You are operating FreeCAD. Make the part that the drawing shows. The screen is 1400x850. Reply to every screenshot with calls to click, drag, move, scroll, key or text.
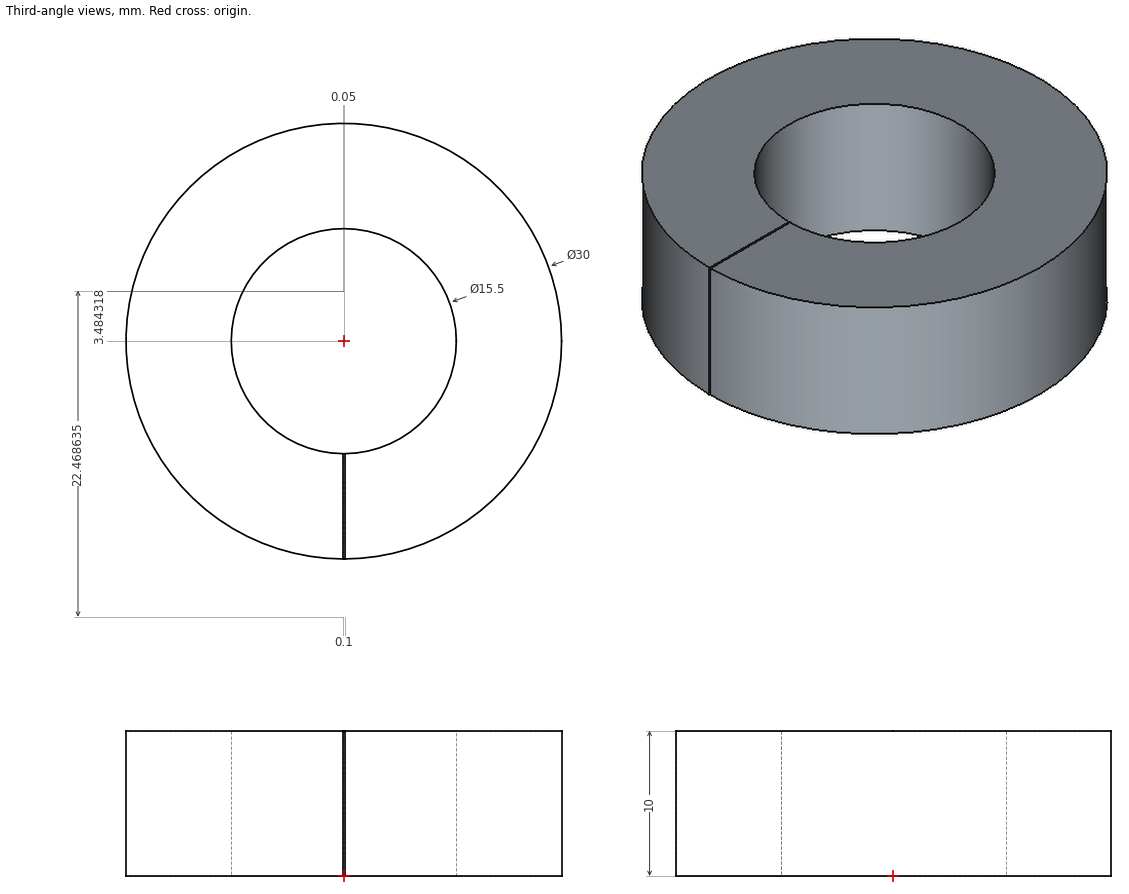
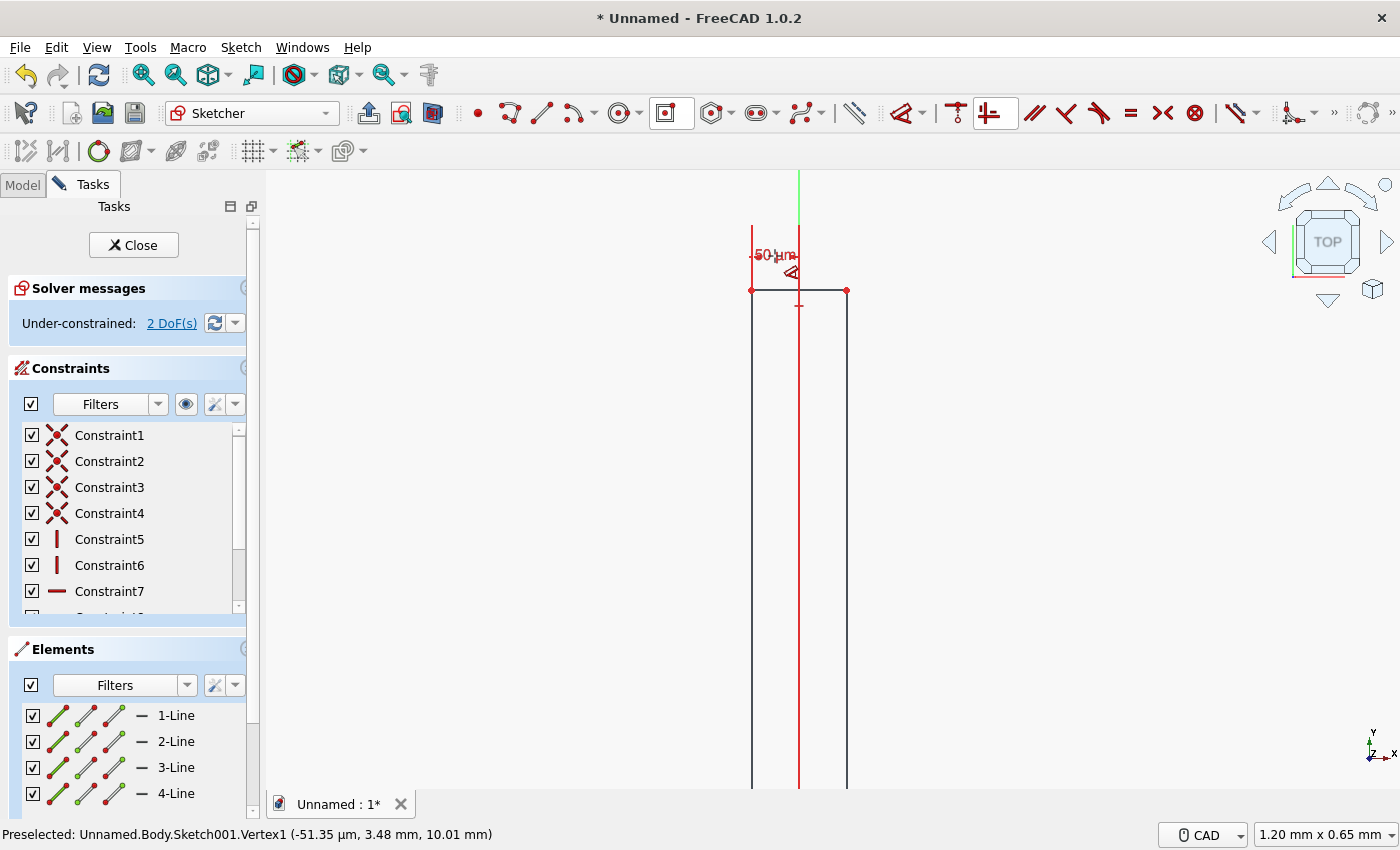
scroll(764, 480, down, 15)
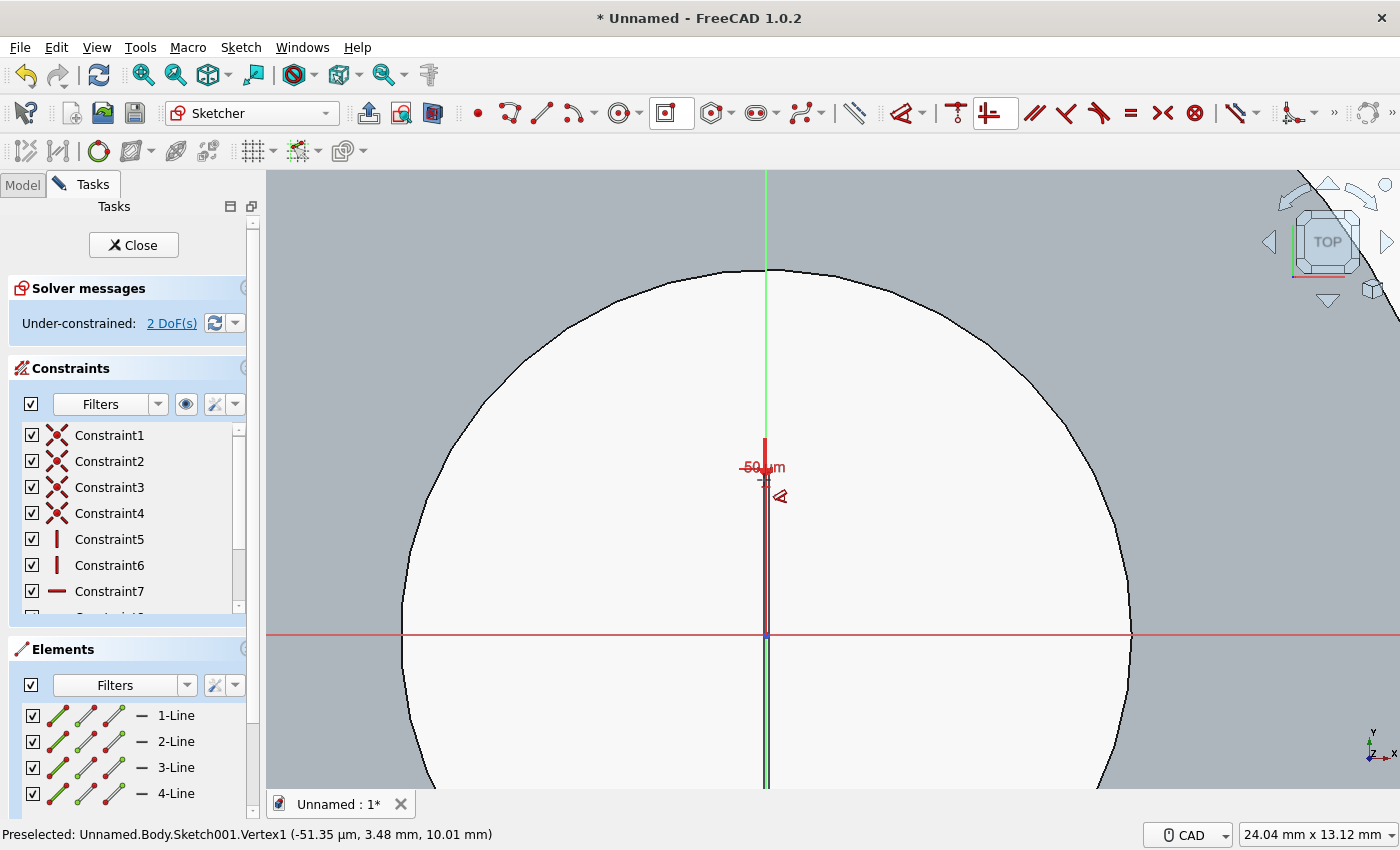
scroll(764, 198, down, 5)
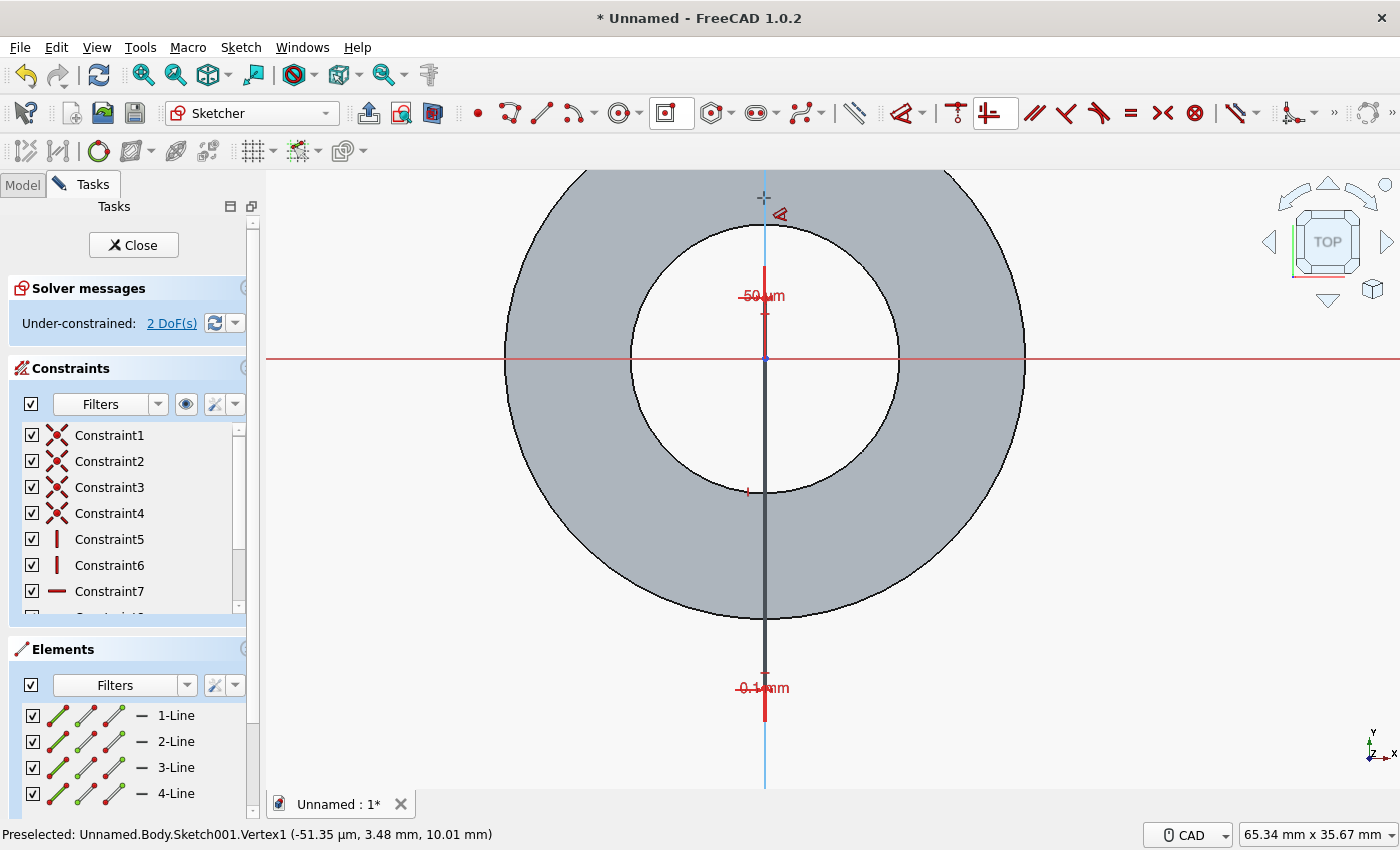
scroll(764, 415, up, 14)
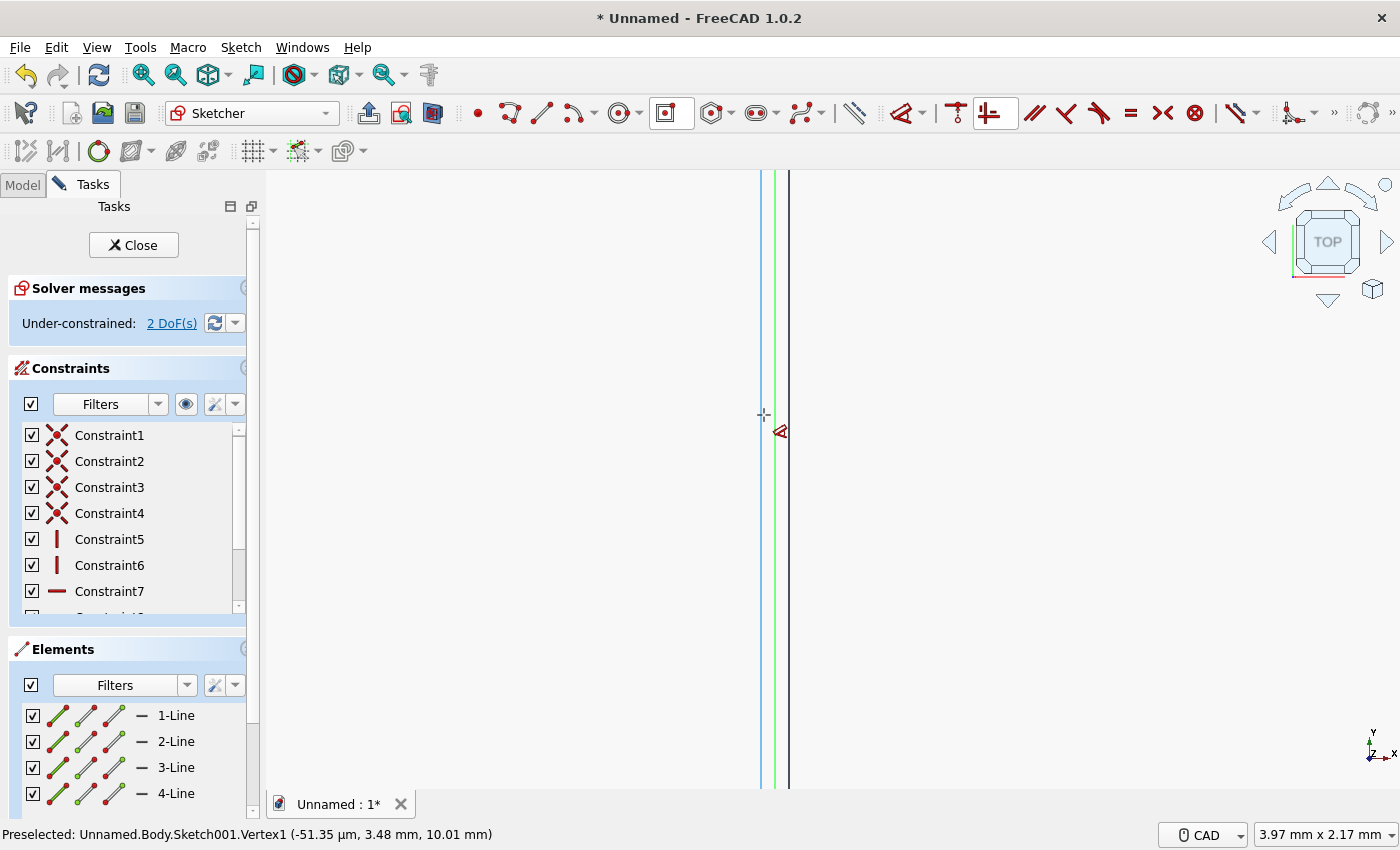
click(761, 416)
click(727, 480)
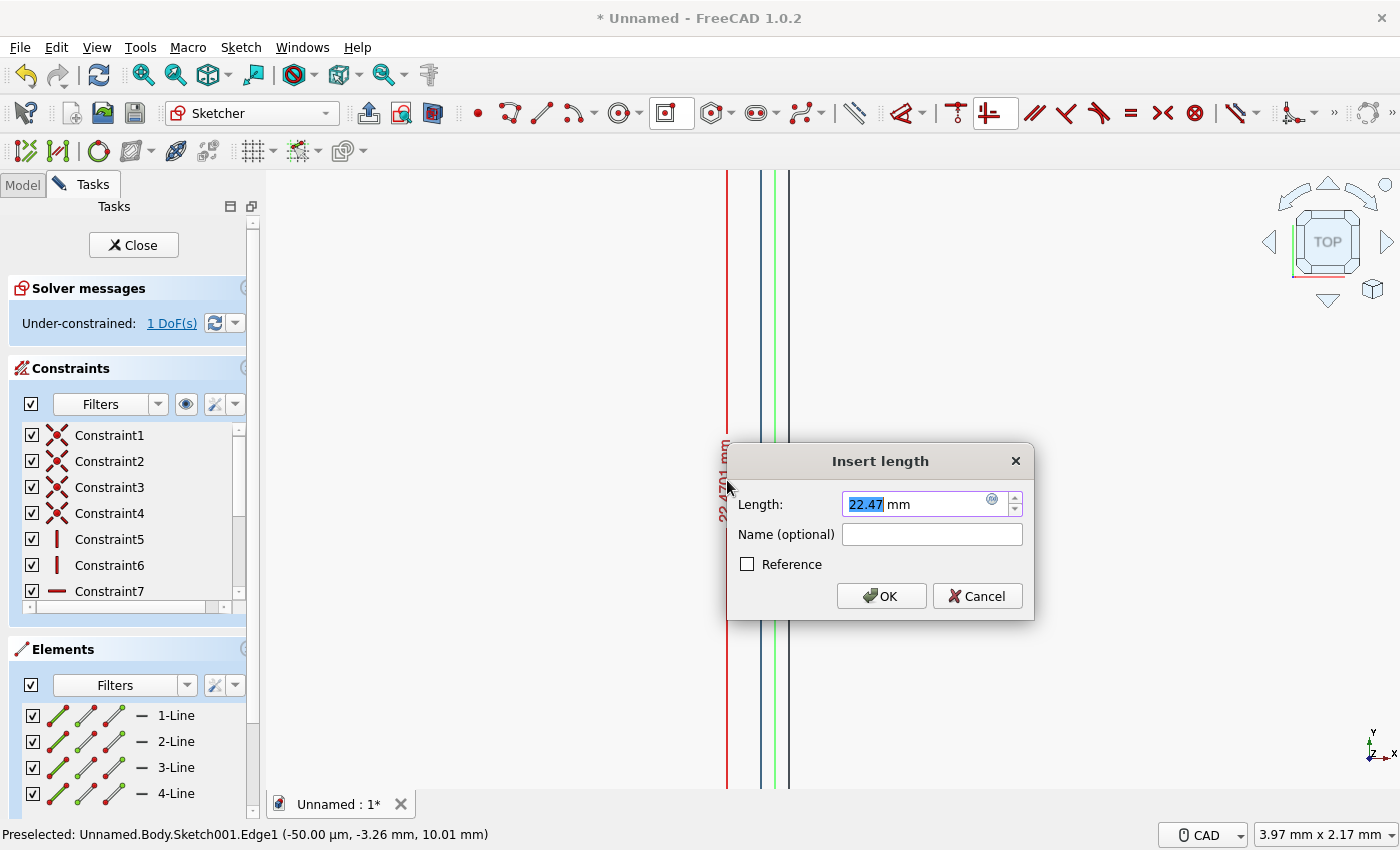
text(22.468635)
key(Return)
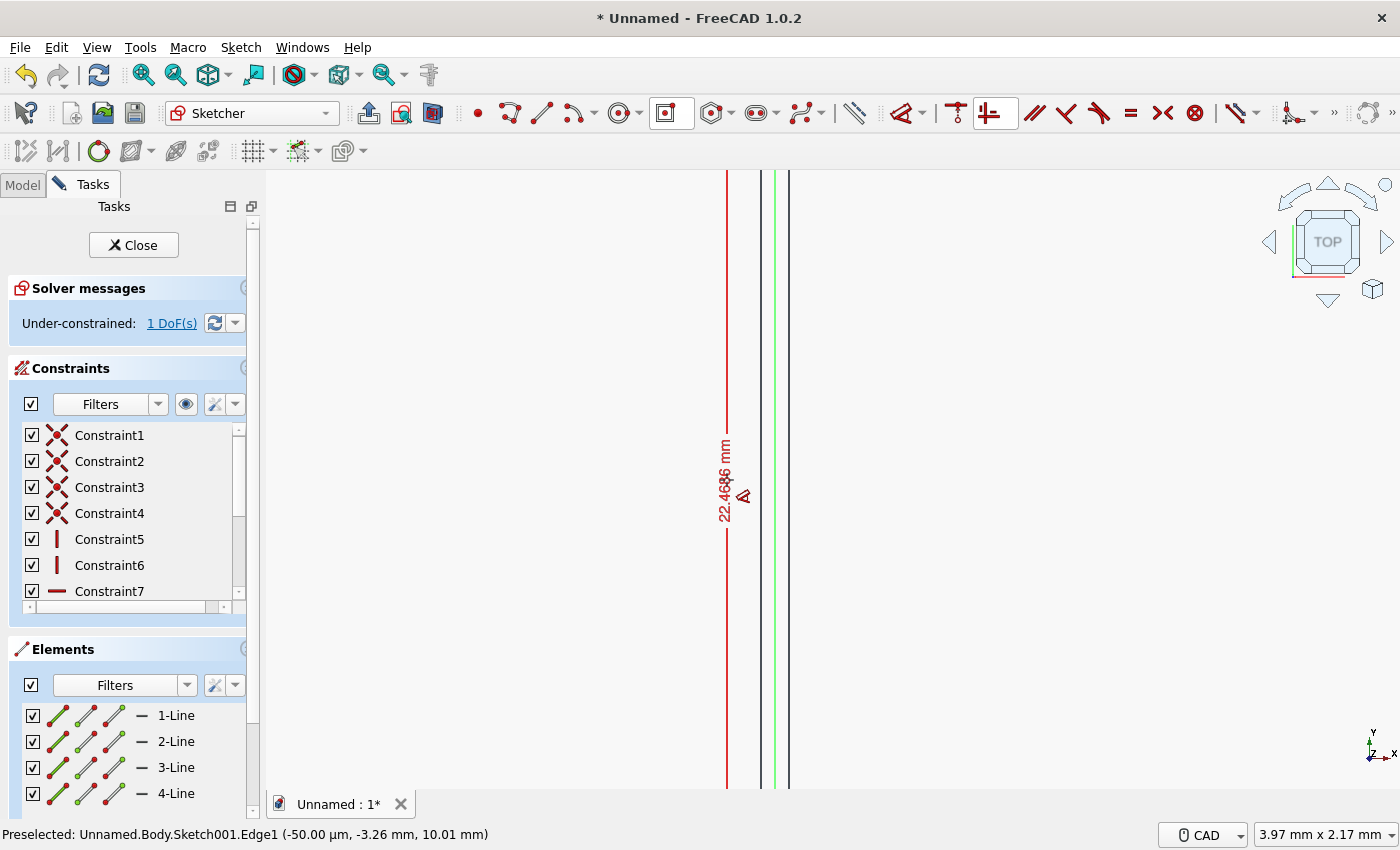
scroll(764, 401, down, 14)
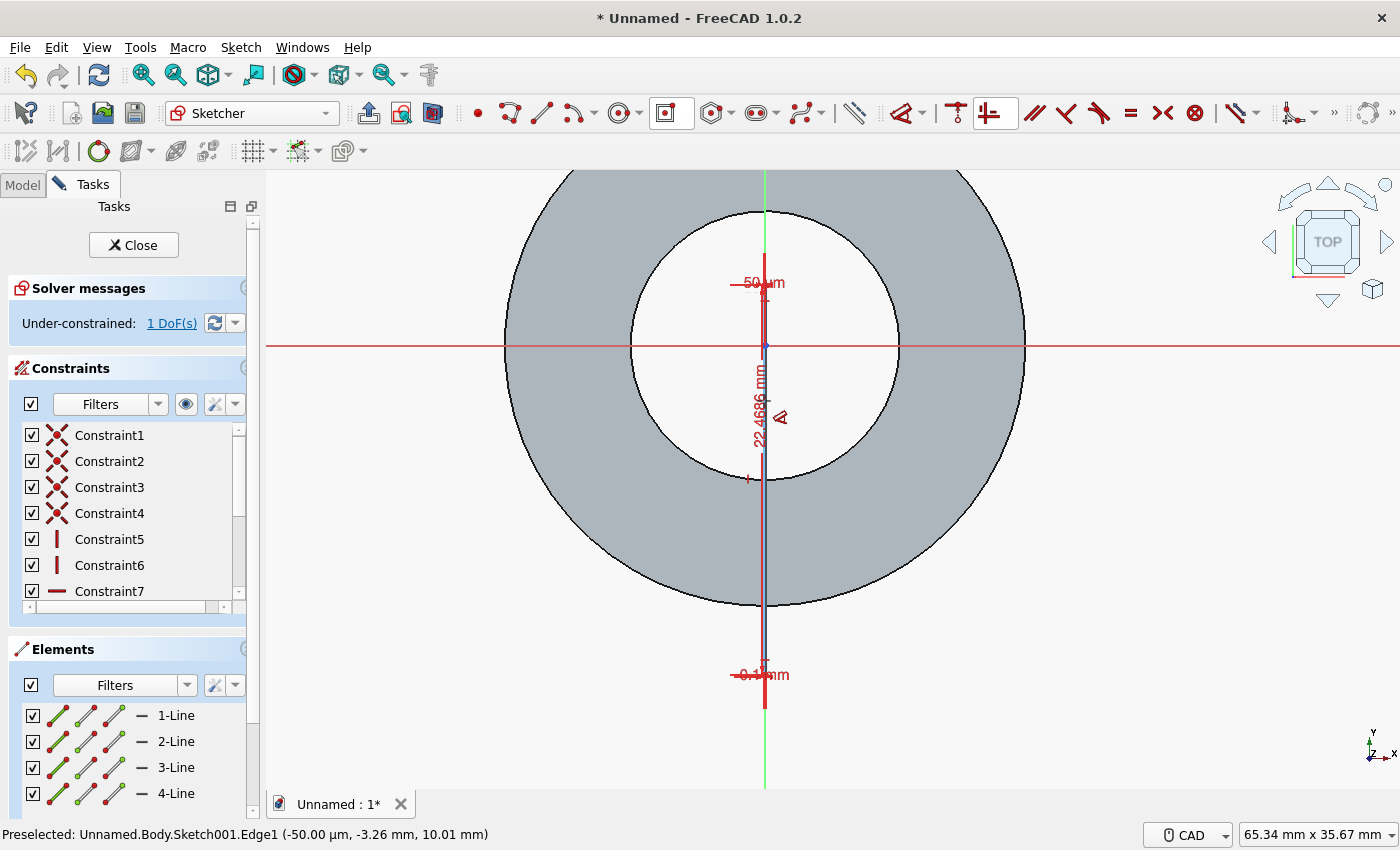
scroll(764, 285, up, 10)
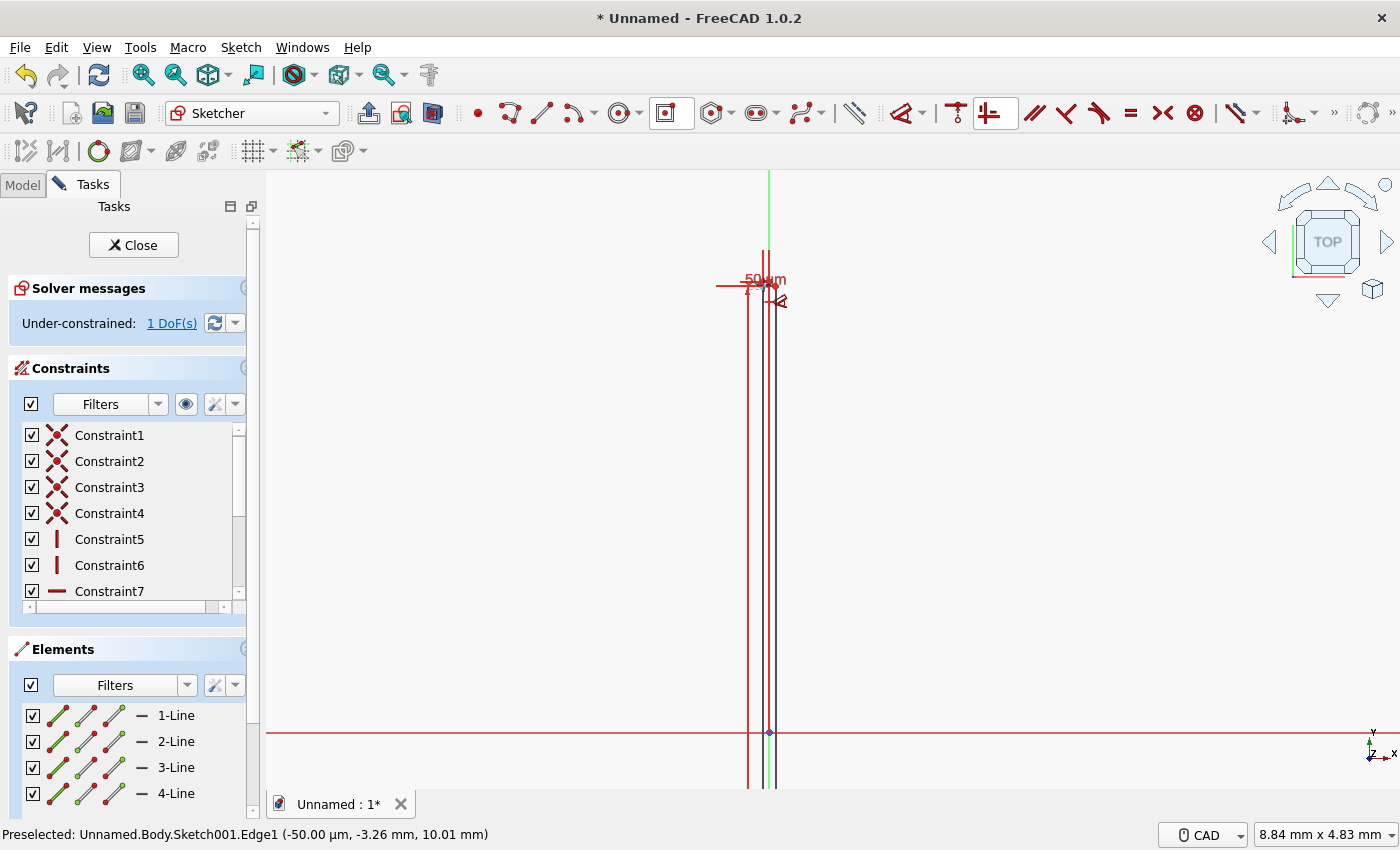
click(763, 286)
click(729, 509)